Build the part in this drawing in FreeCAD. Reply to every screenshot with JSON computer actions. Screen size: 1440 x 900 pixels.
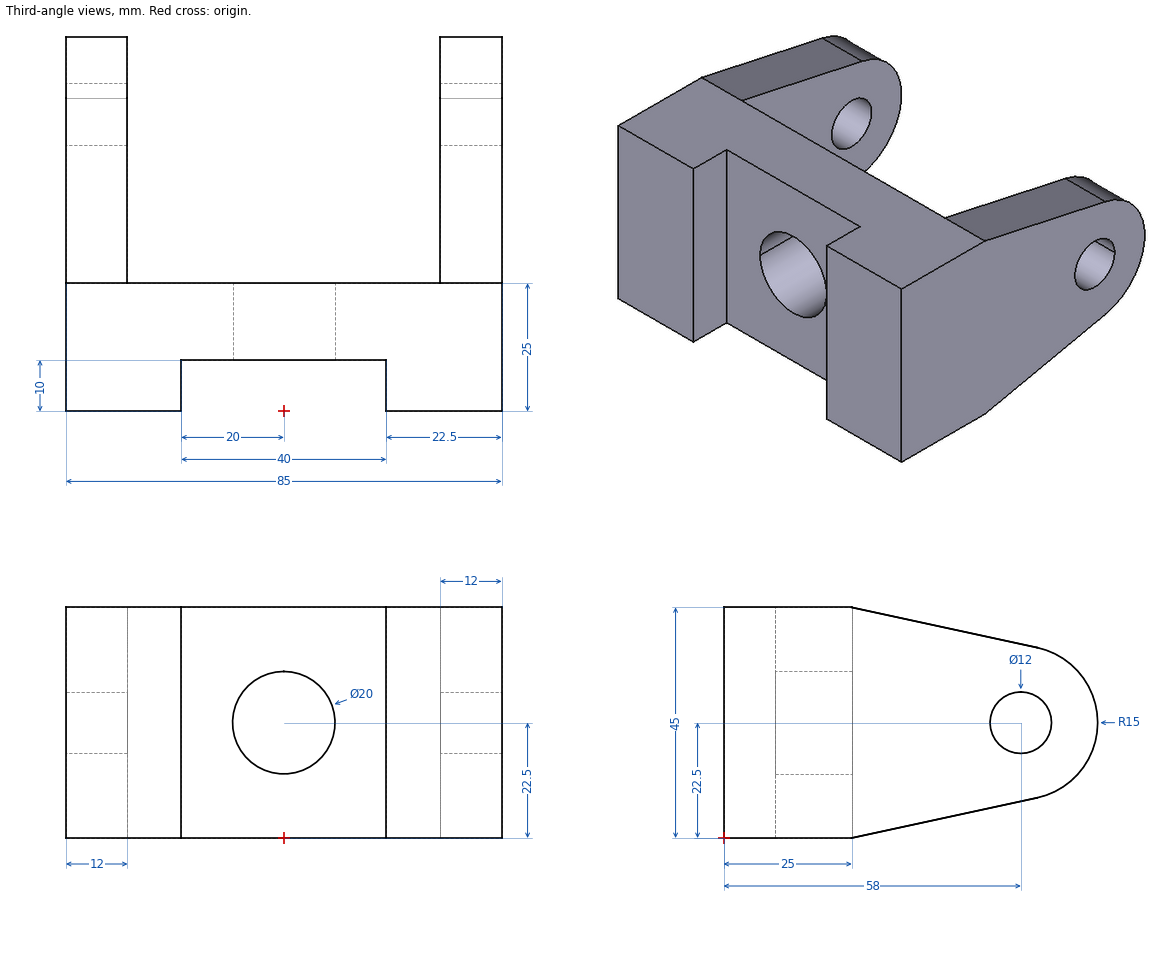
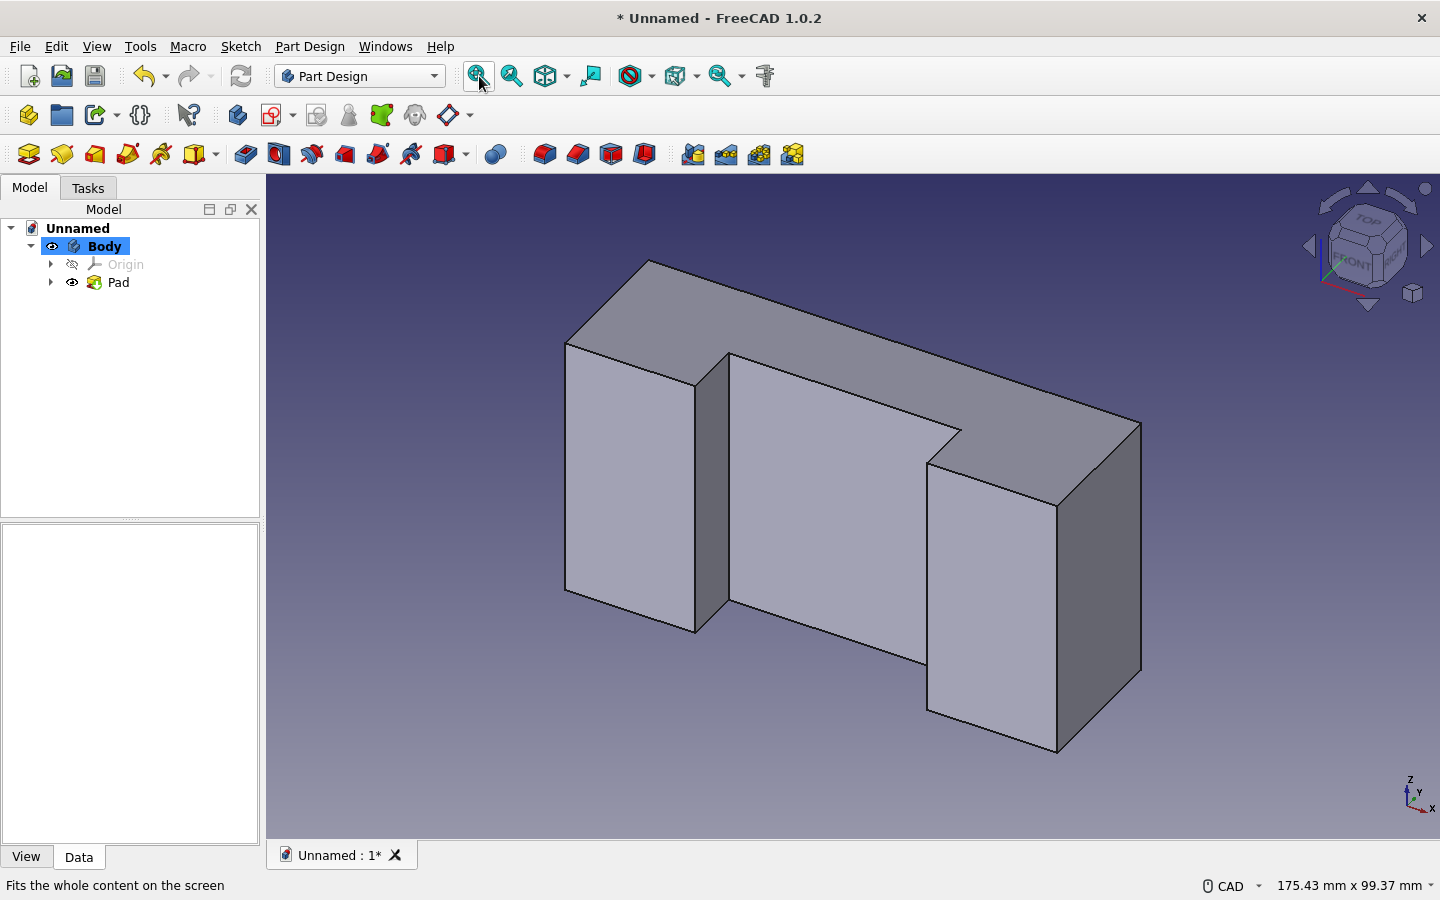
{"action": "key", "text": "4"}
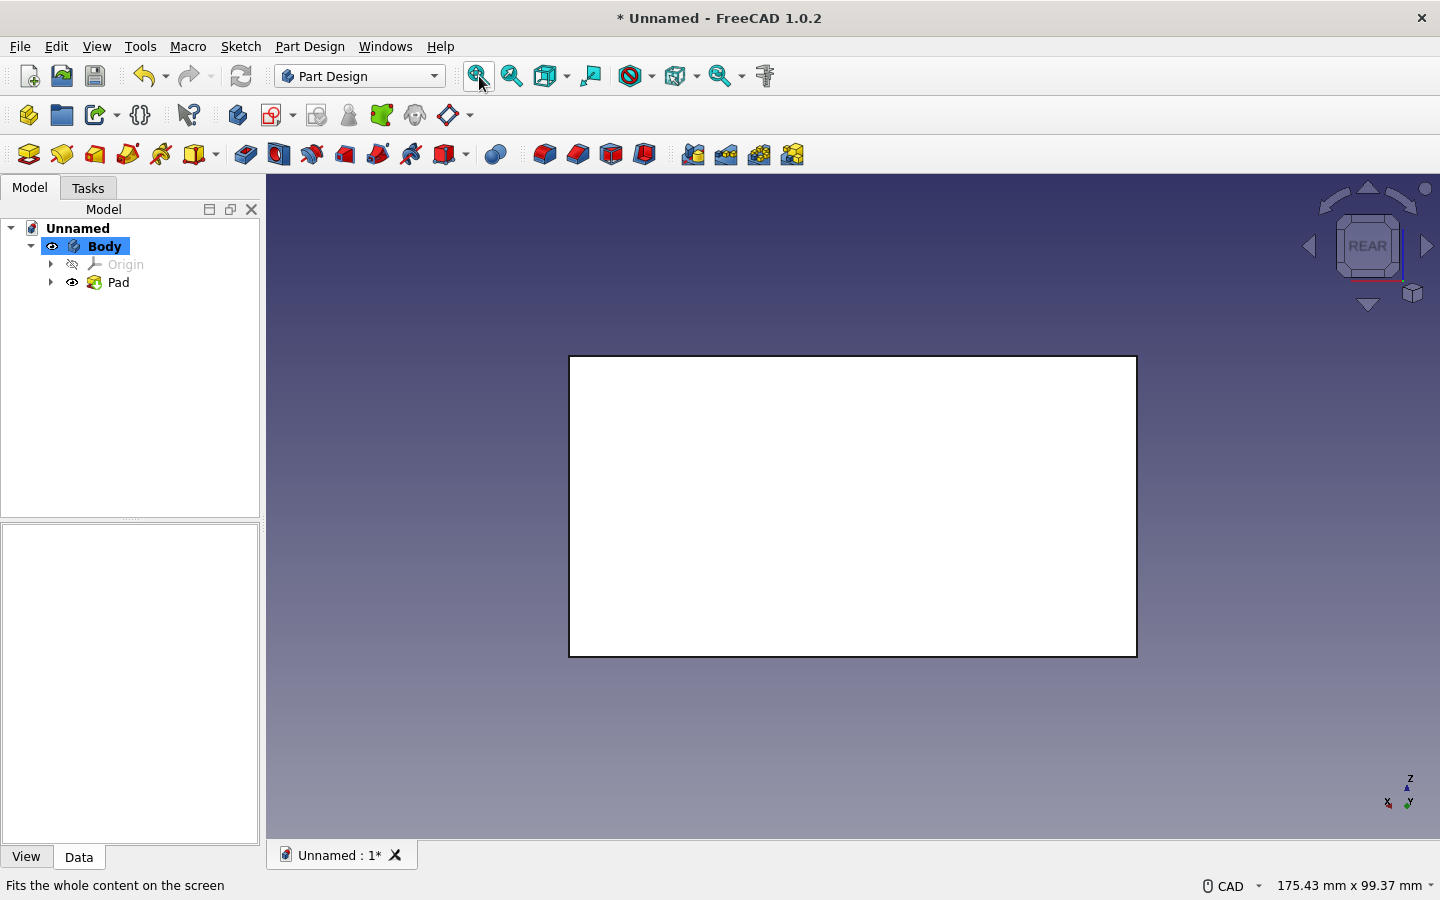
{"action": "left_click", "coordinate": [772, 506]}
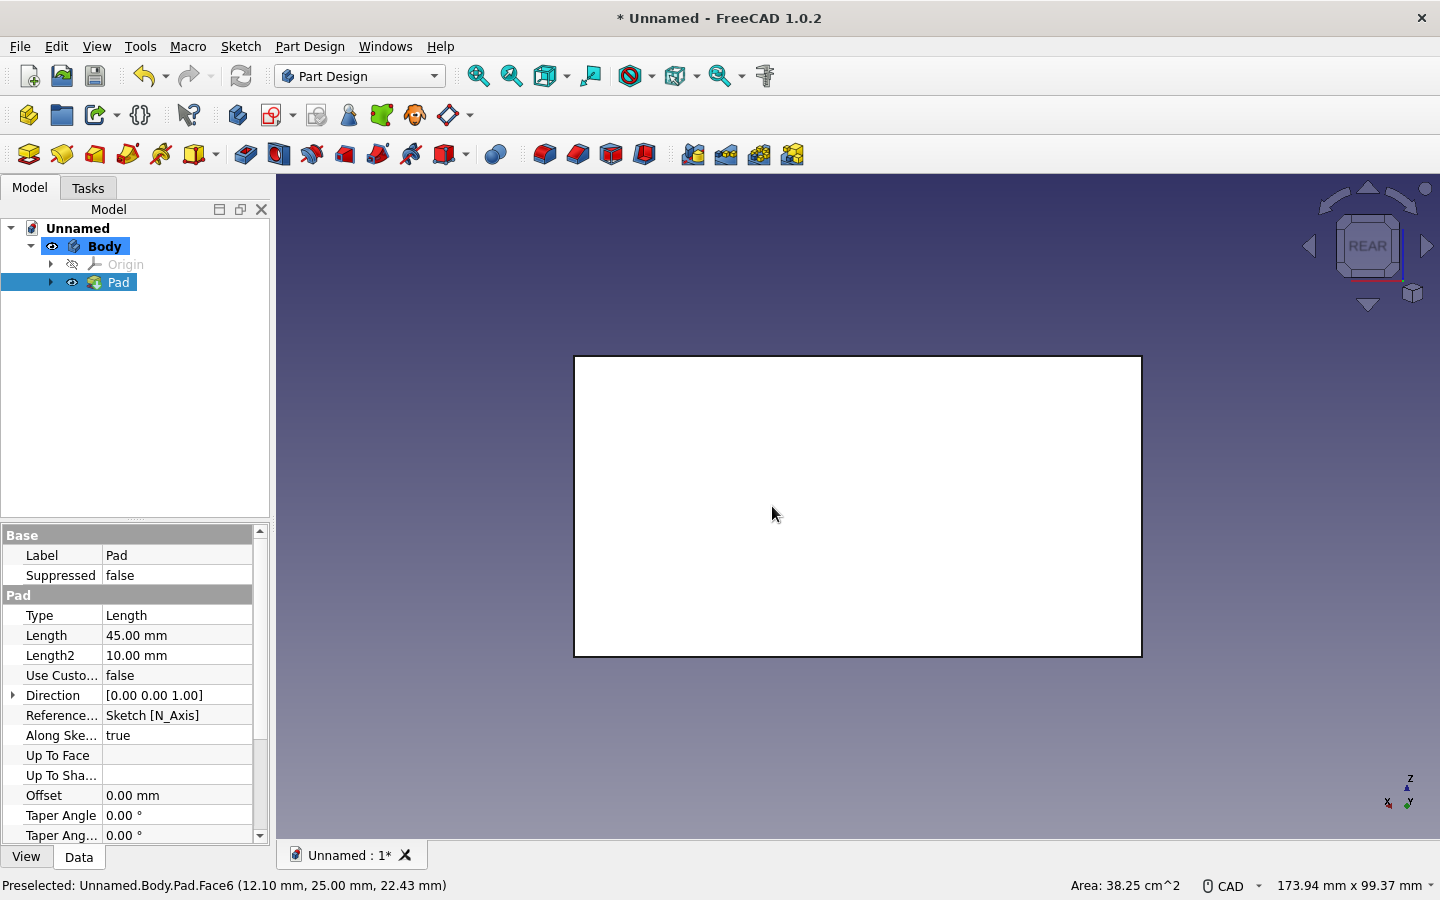
{"action": "left_click", "coordinate": [270, 116]}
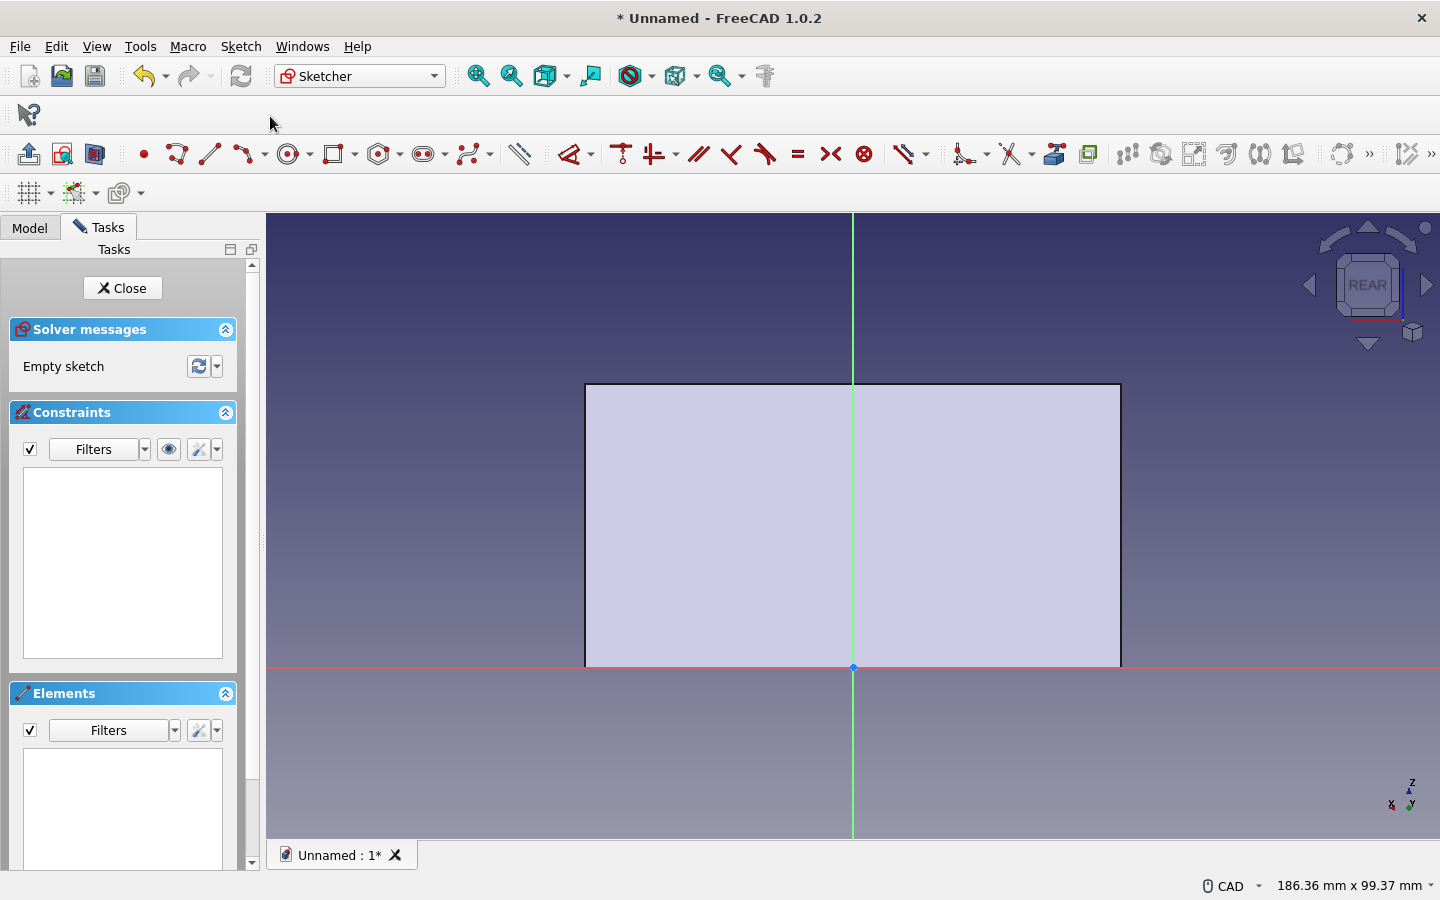
{"action": "scroll", "coordinate": [936, 613], "scroll_direction": "up", "scroll_amount": 3}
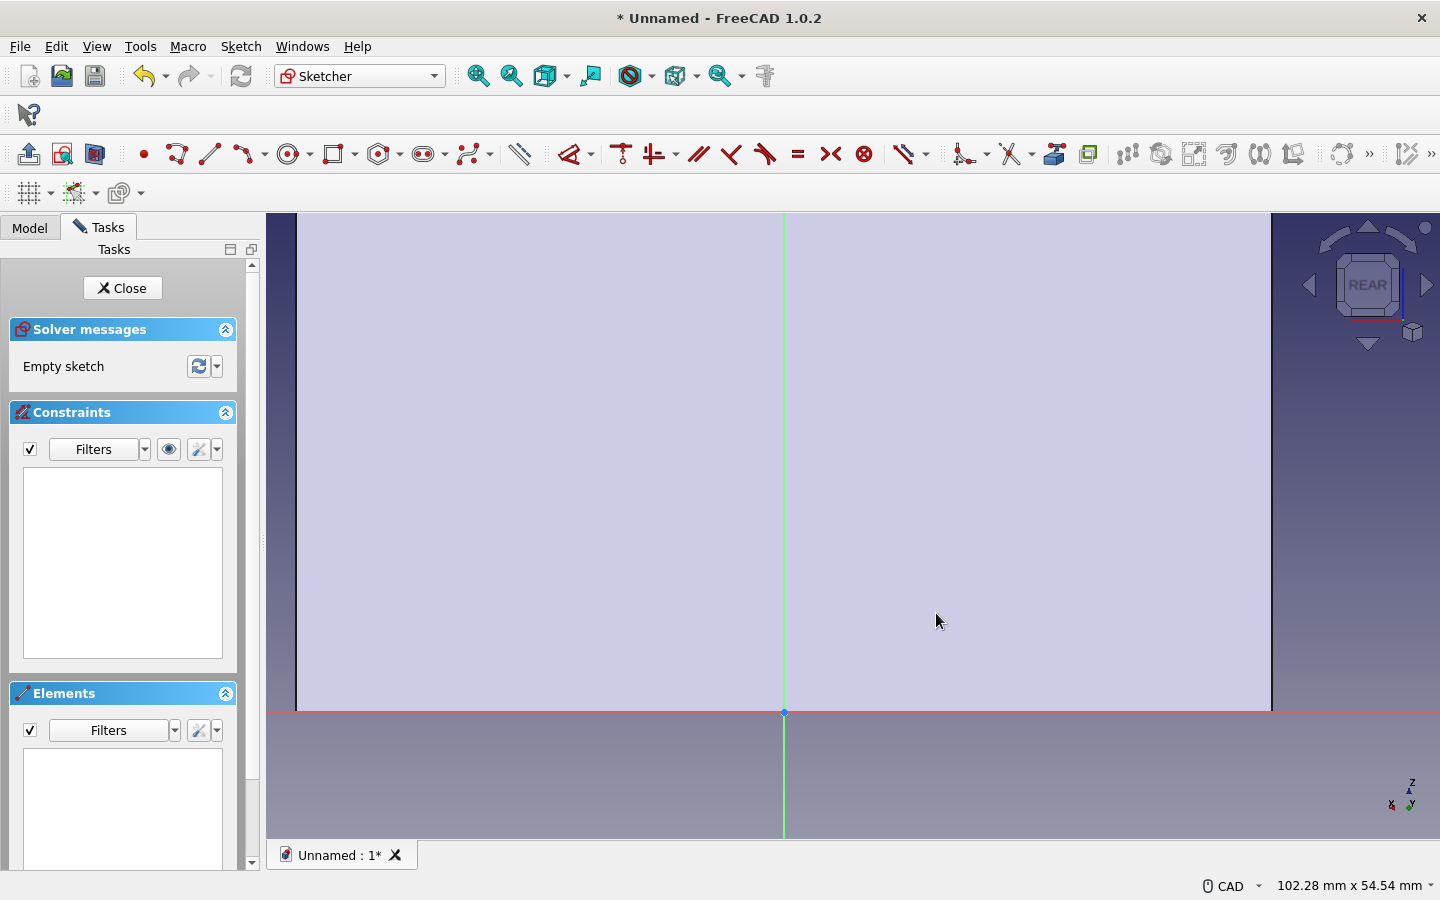
{"action": "left_click", "coordinate": [288, 154]}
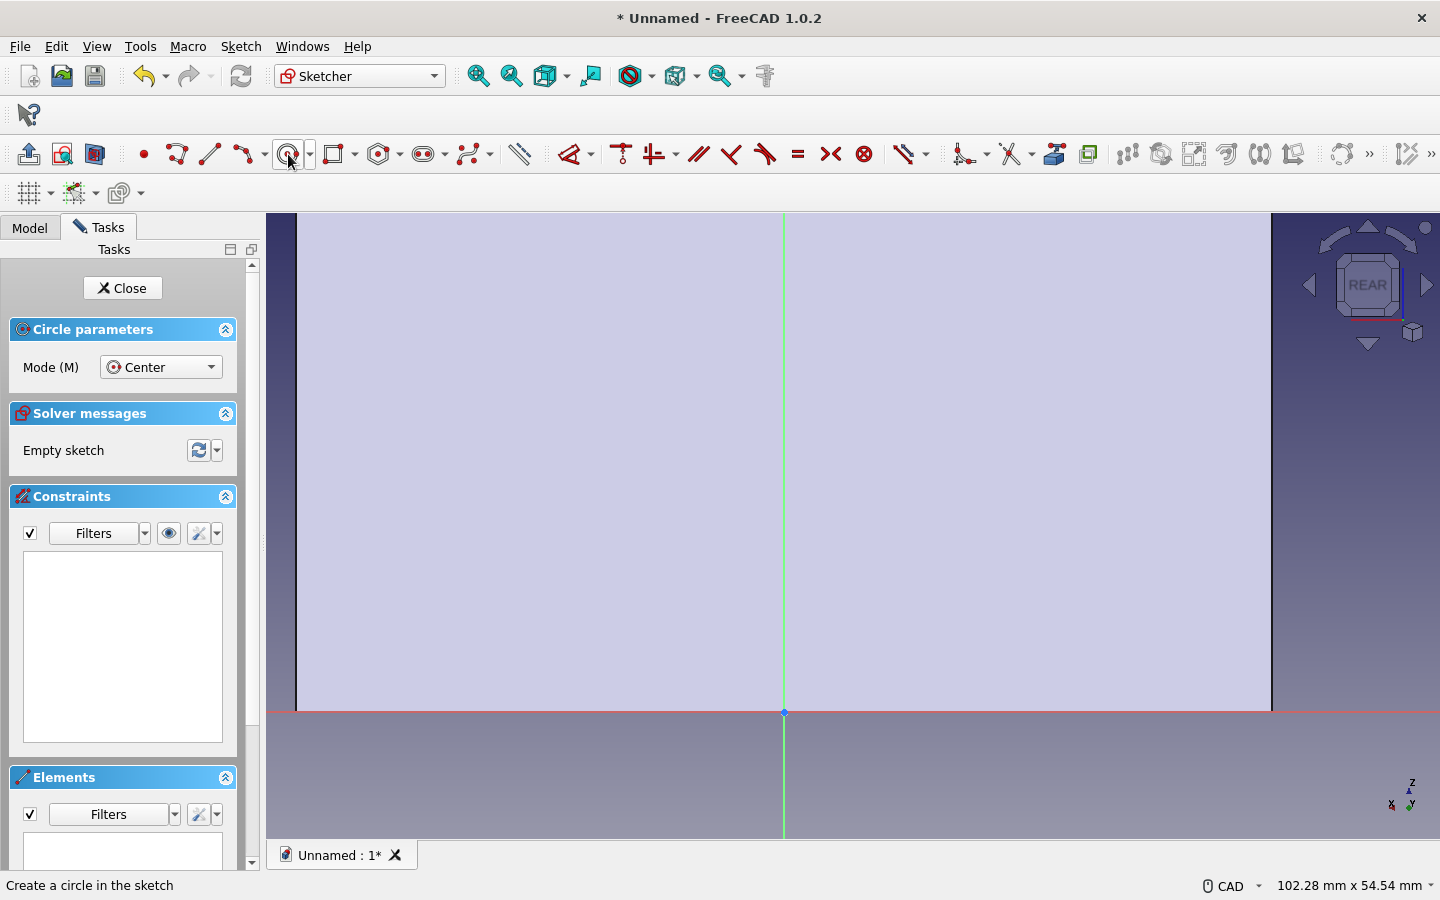
{"action": "left_click", "coordinate": [784, 454]}
{"action": "mouse_move", "coordinate": [865, 373]}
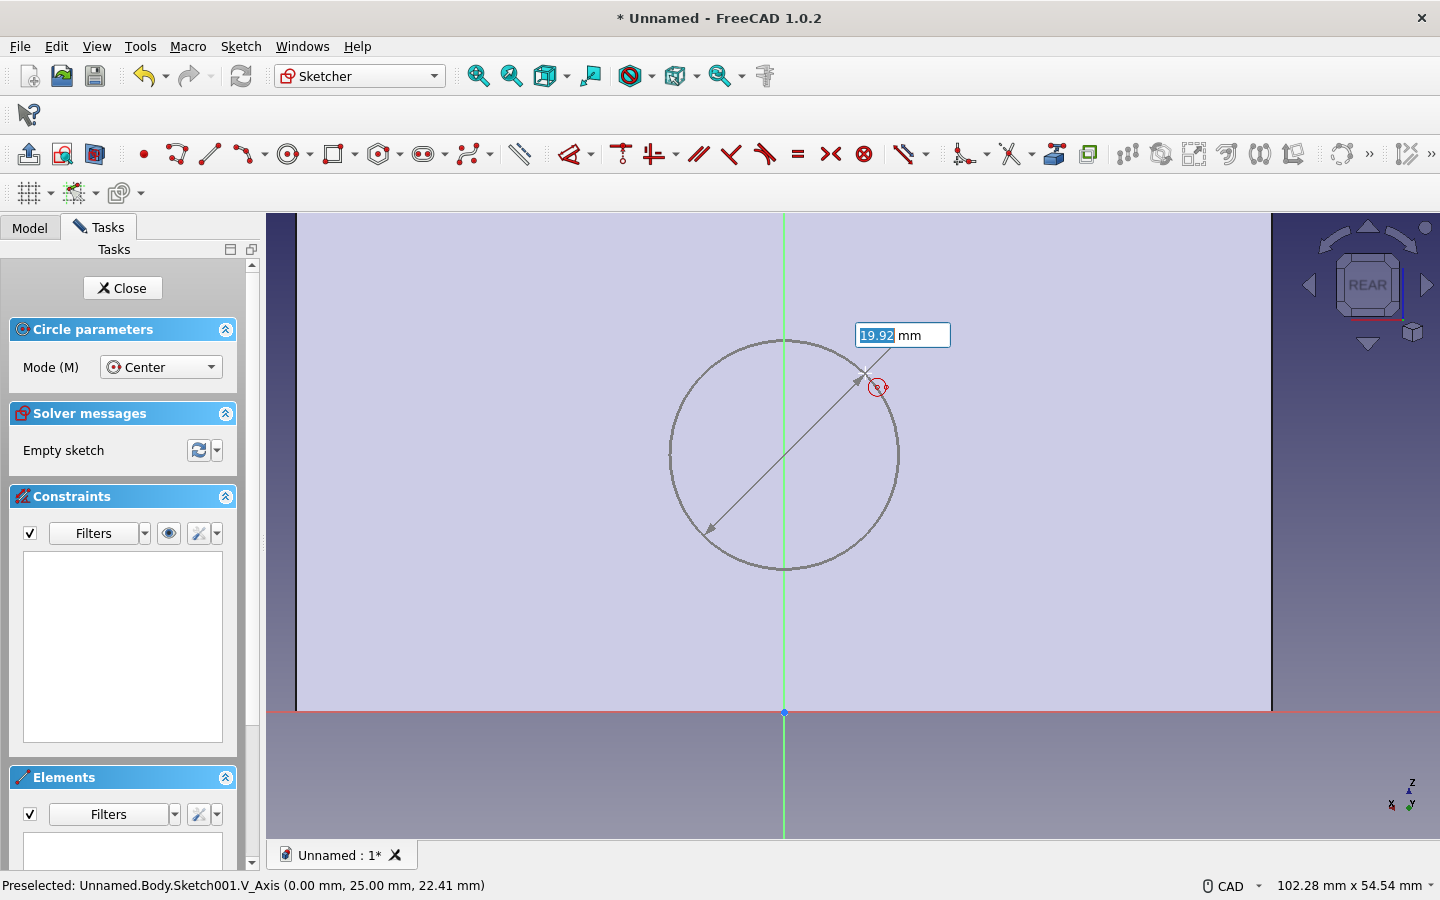
{"action": "type", "text": "20"}
{"action": "key", "text": "Return"}
{"action": "key", "text": "Escape"}